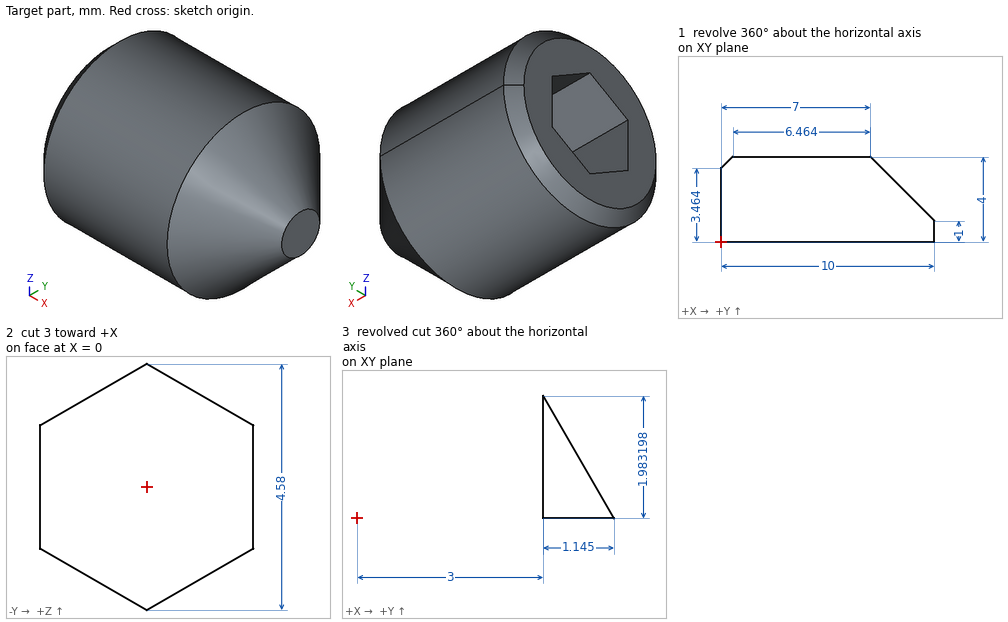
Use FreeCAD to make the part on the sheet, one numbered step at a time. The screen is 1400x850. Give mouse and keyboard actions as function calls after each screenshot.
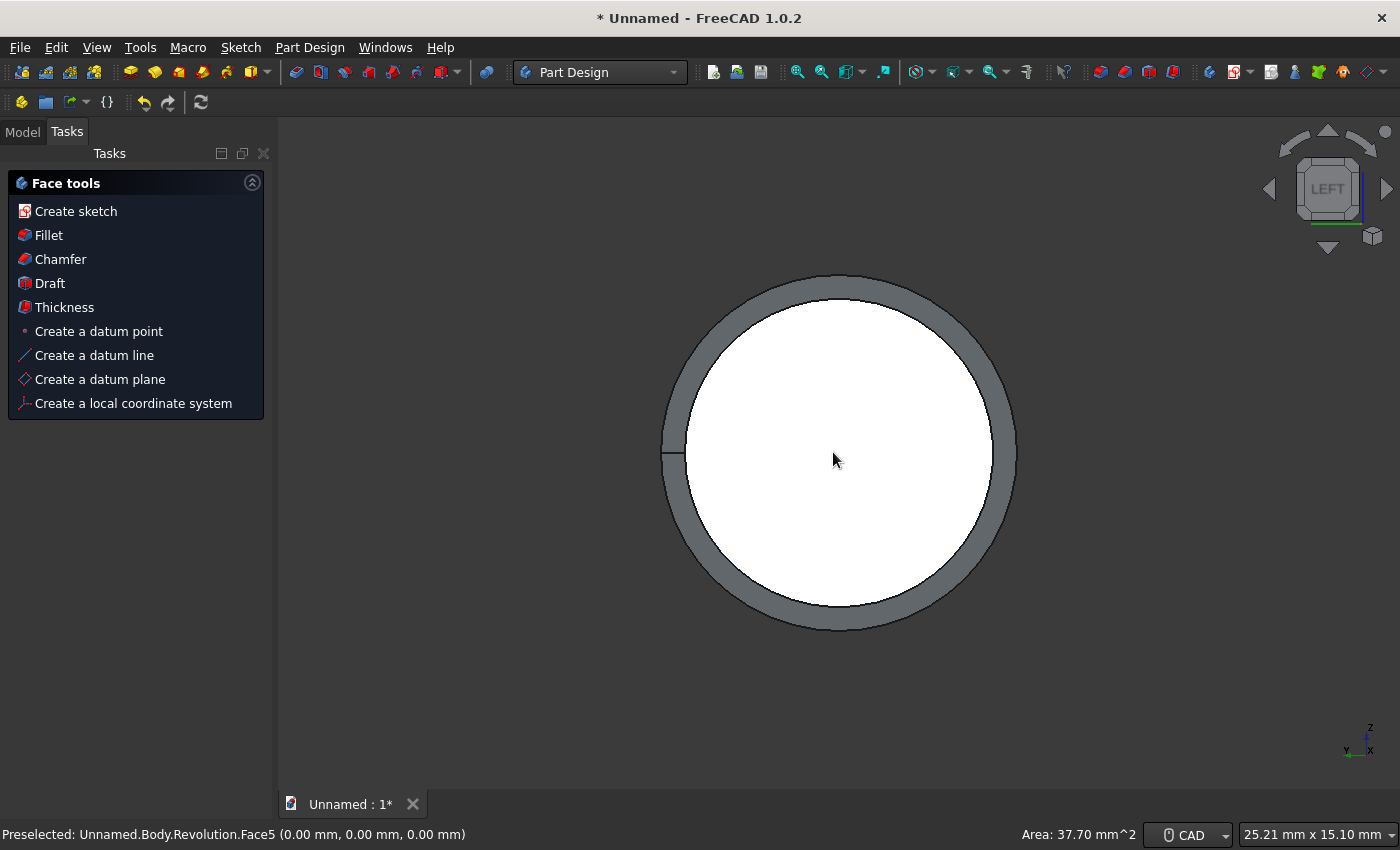
click(1234, 72)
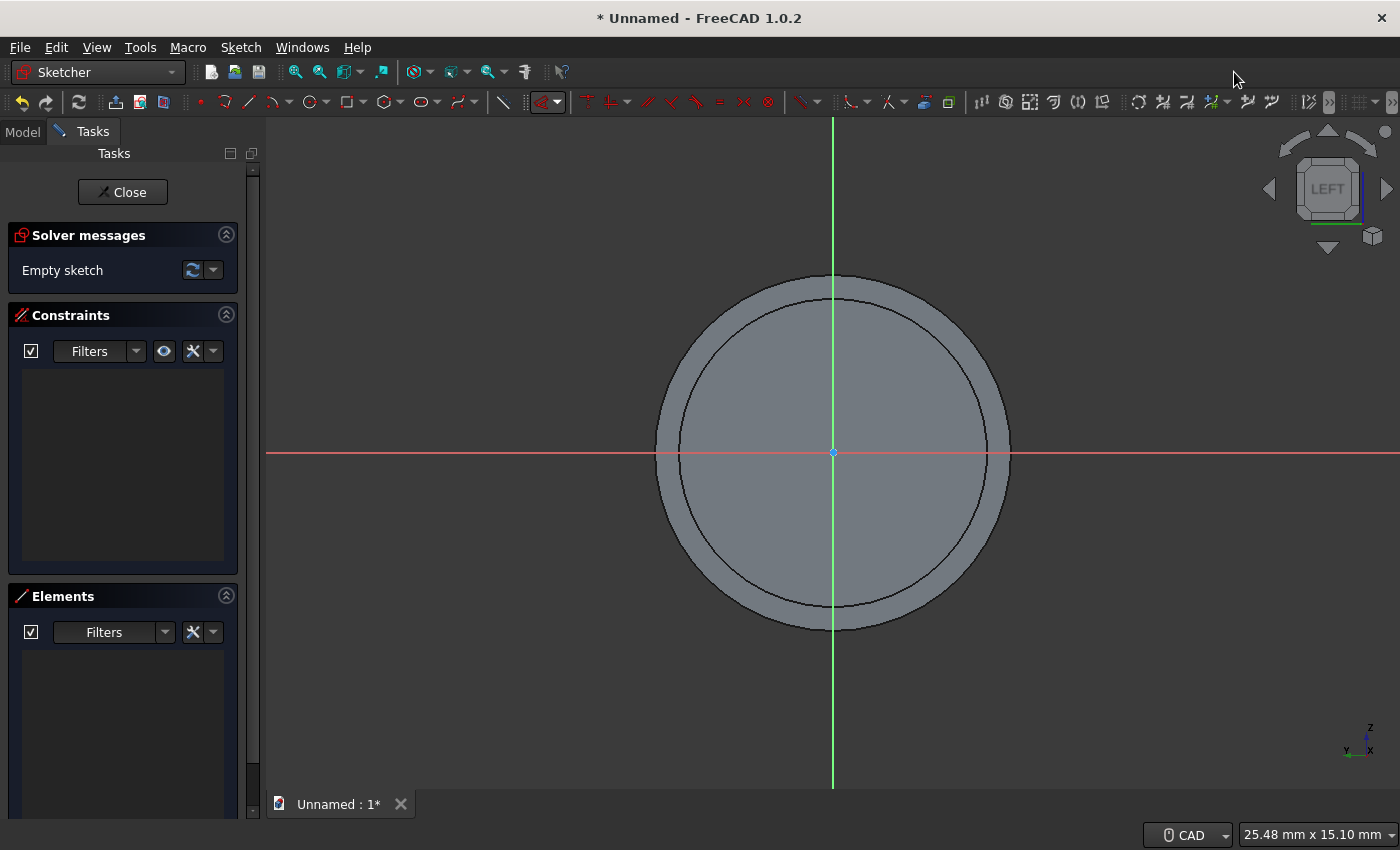
scroll(889, 453, up, 4)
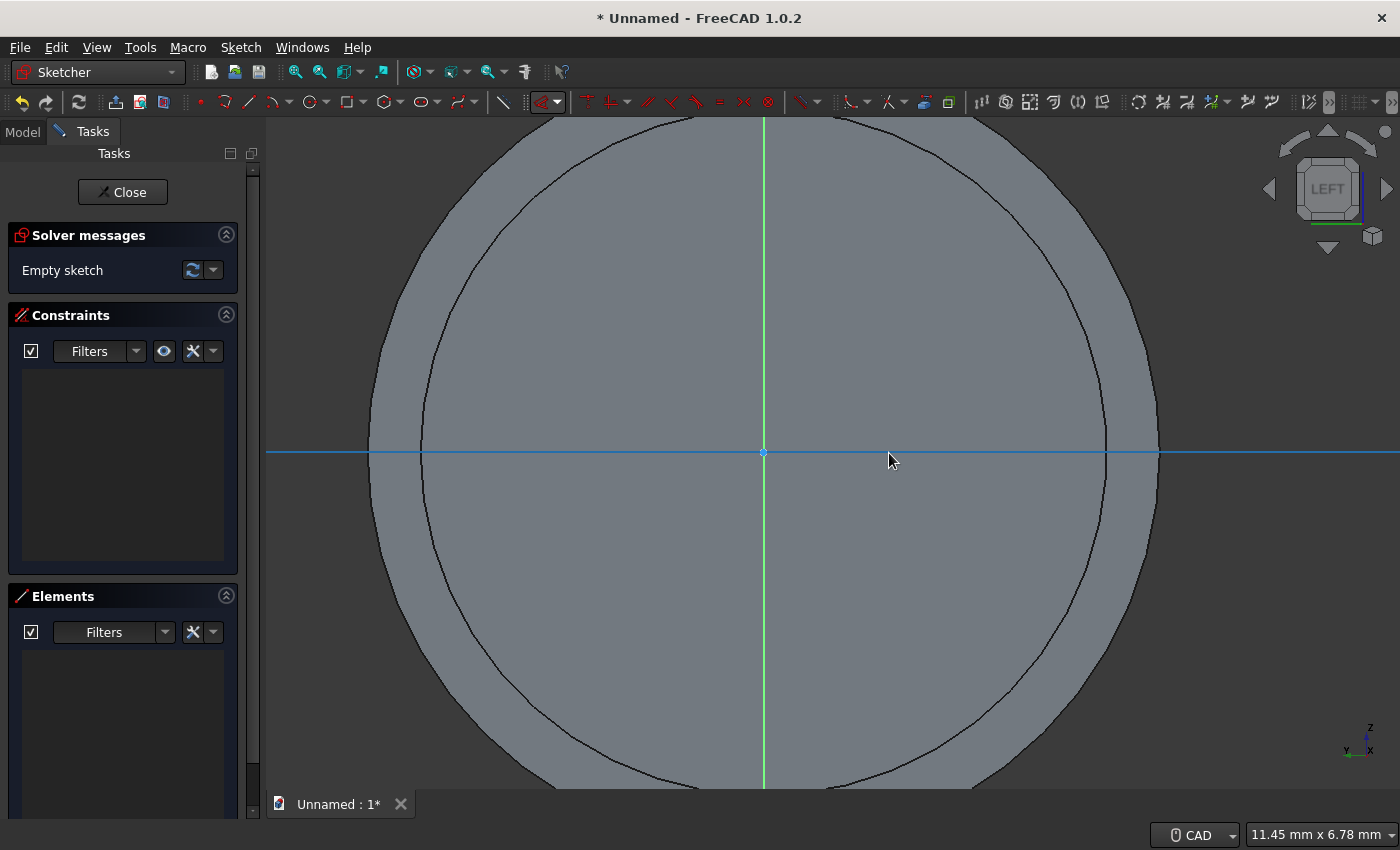
click(384, 102)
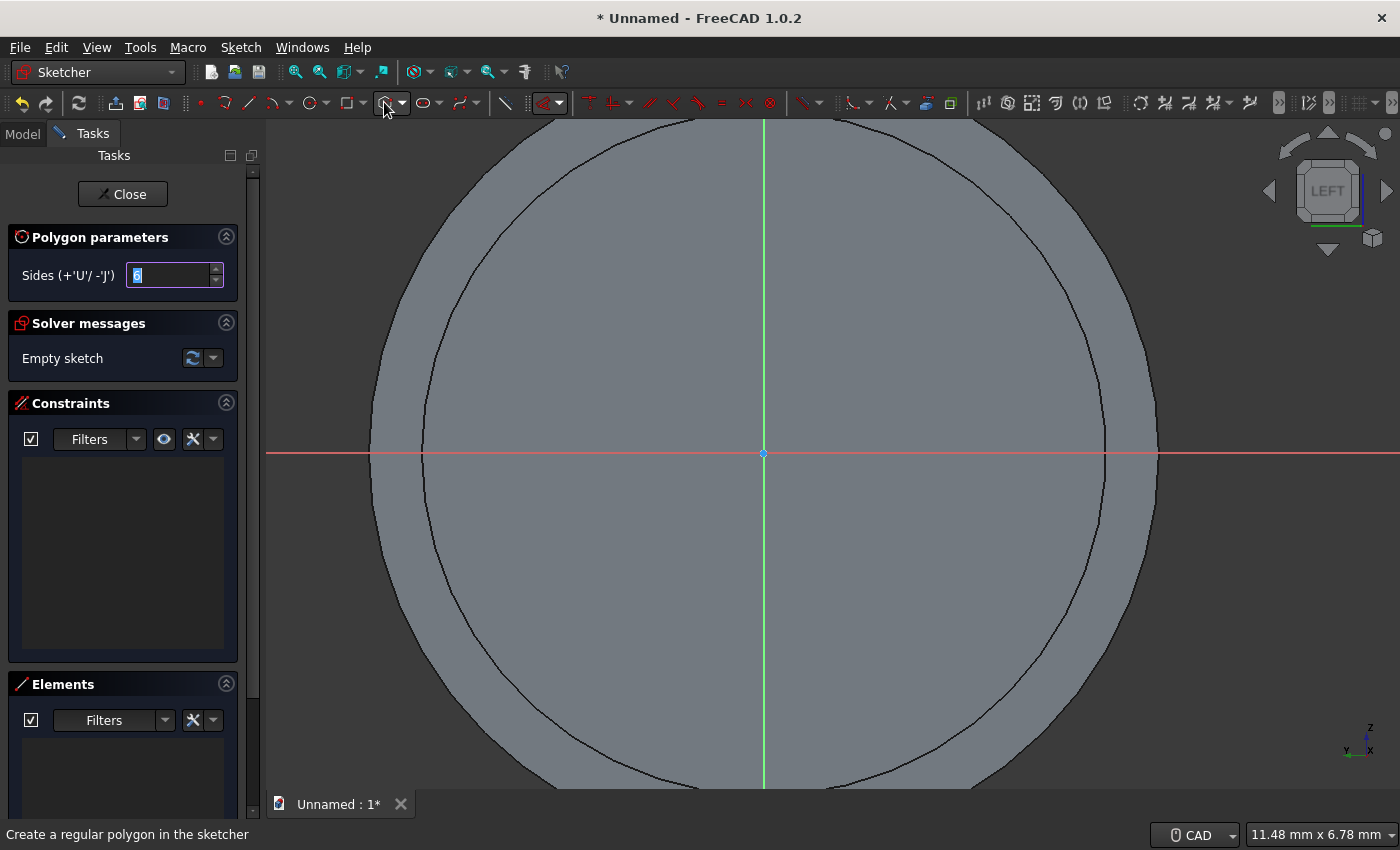
click(764, 453)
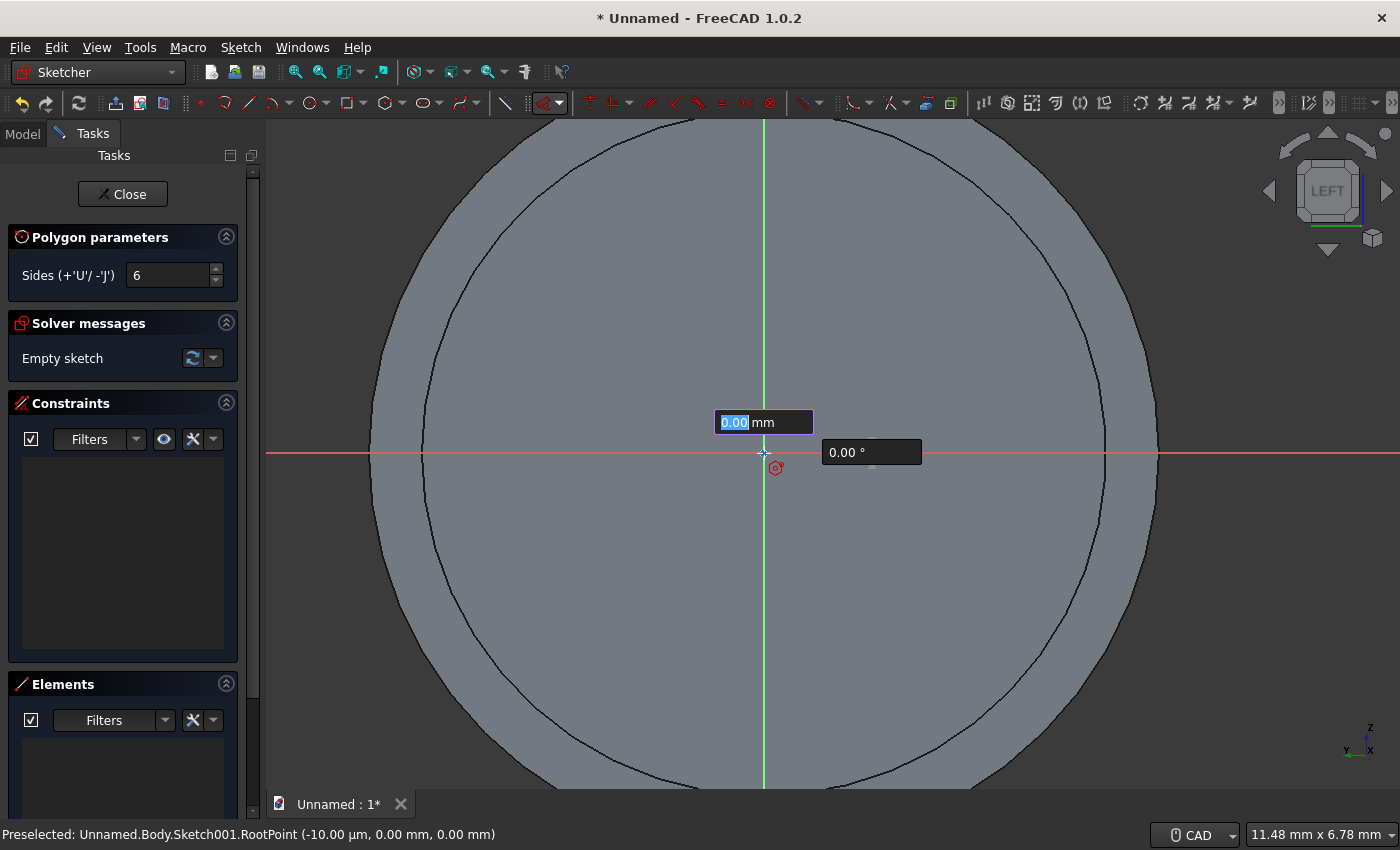
click(764, 227)
right_click(764, 227)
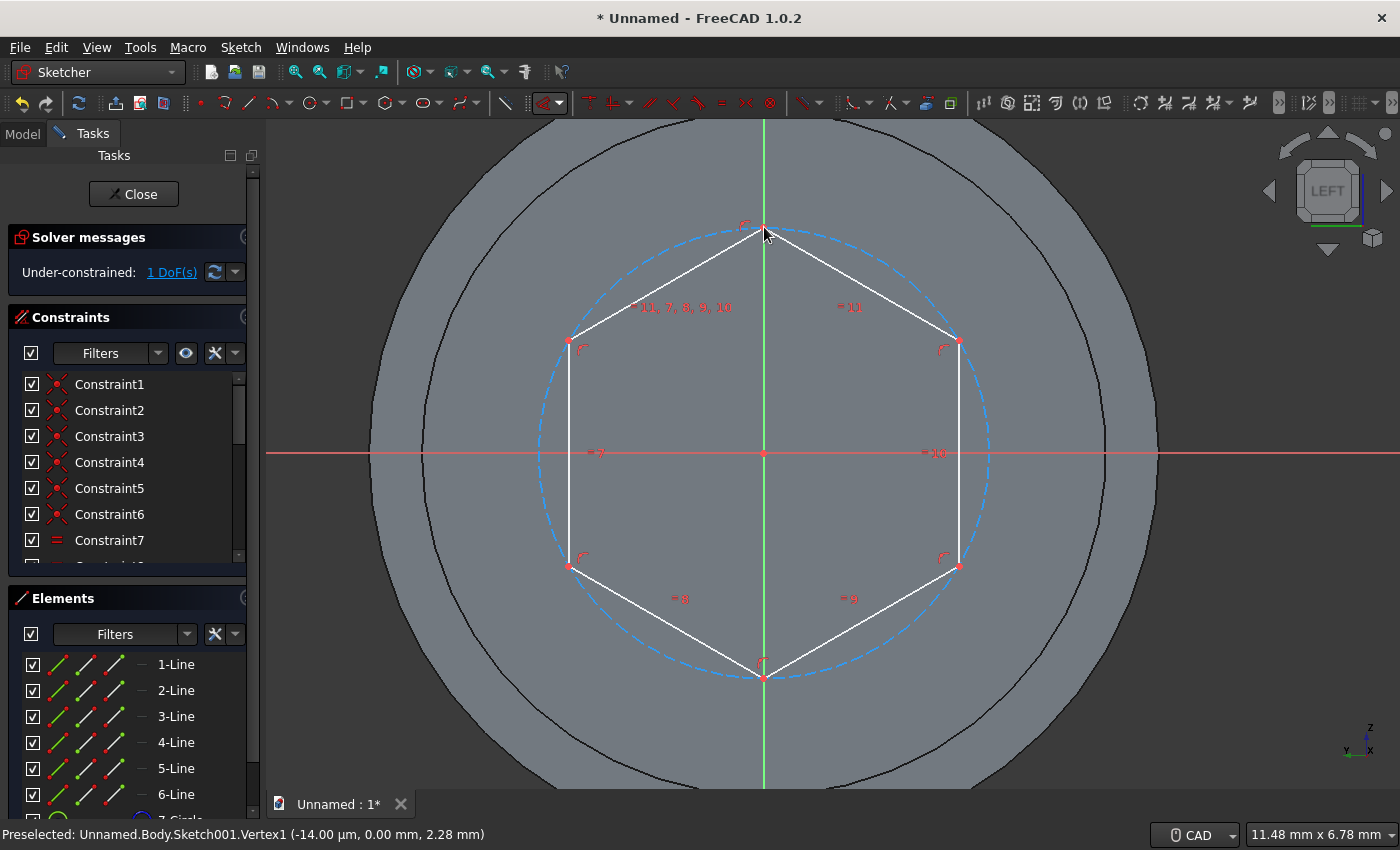
click(764, 679)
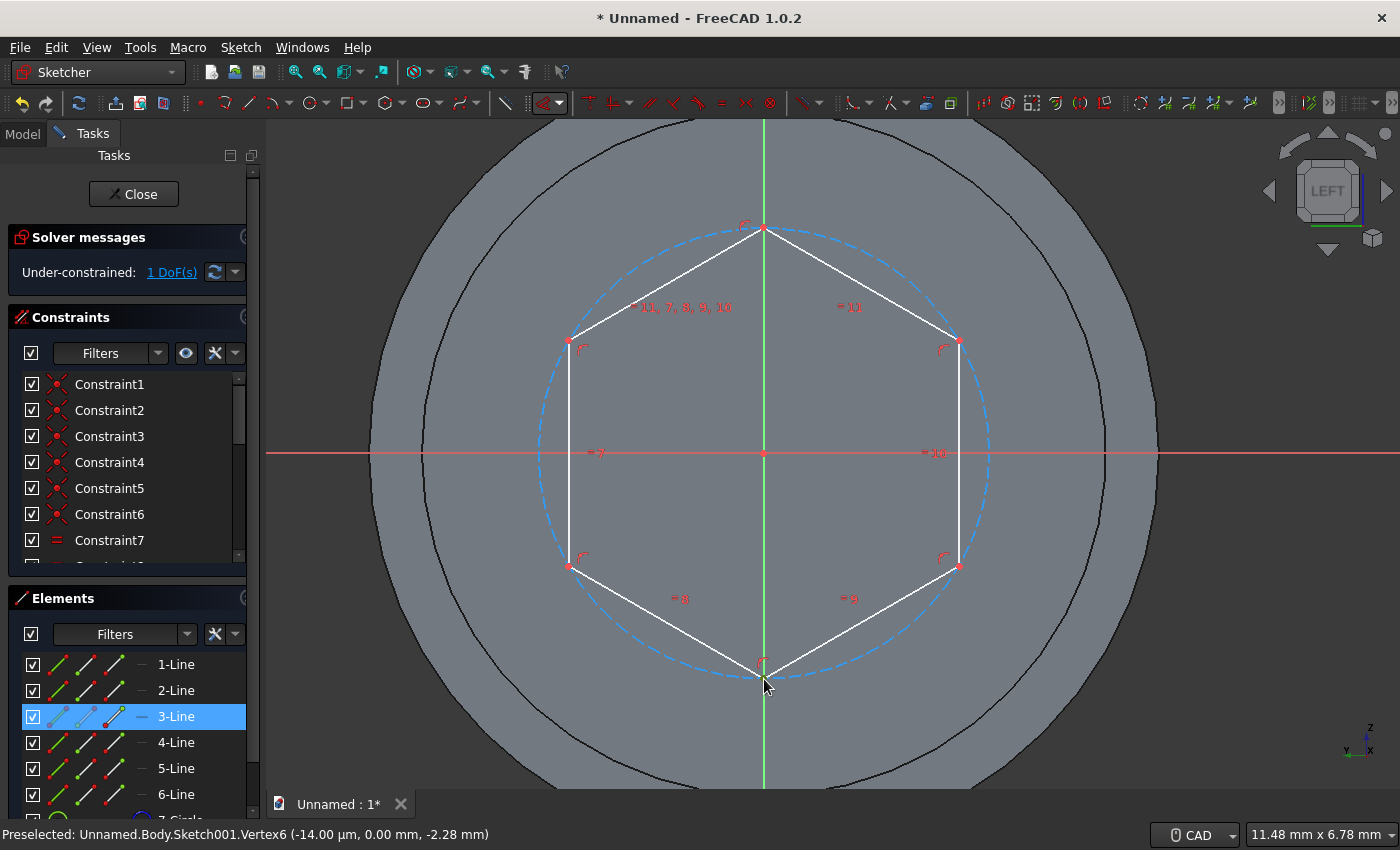
click(764, 228)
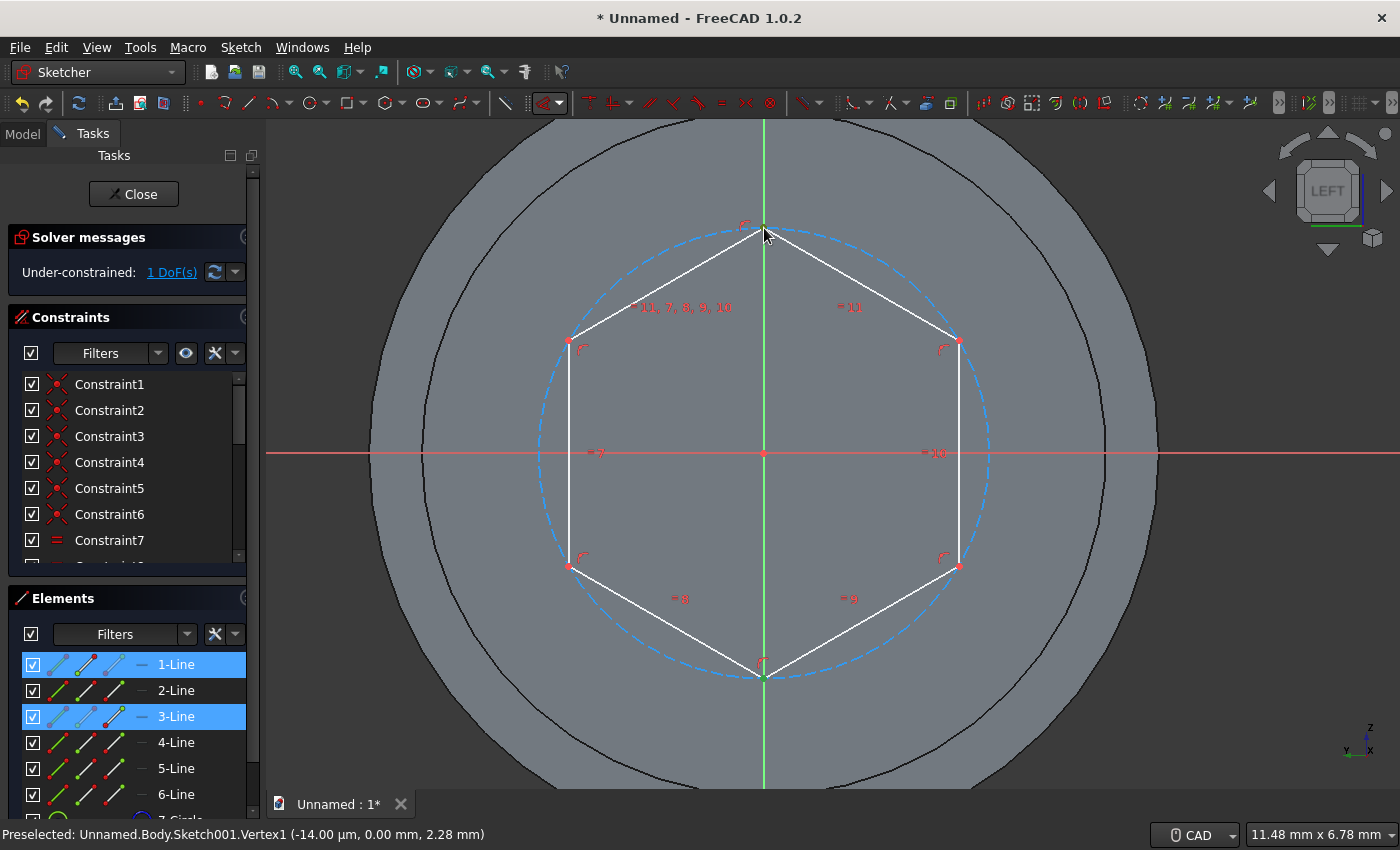
key(i)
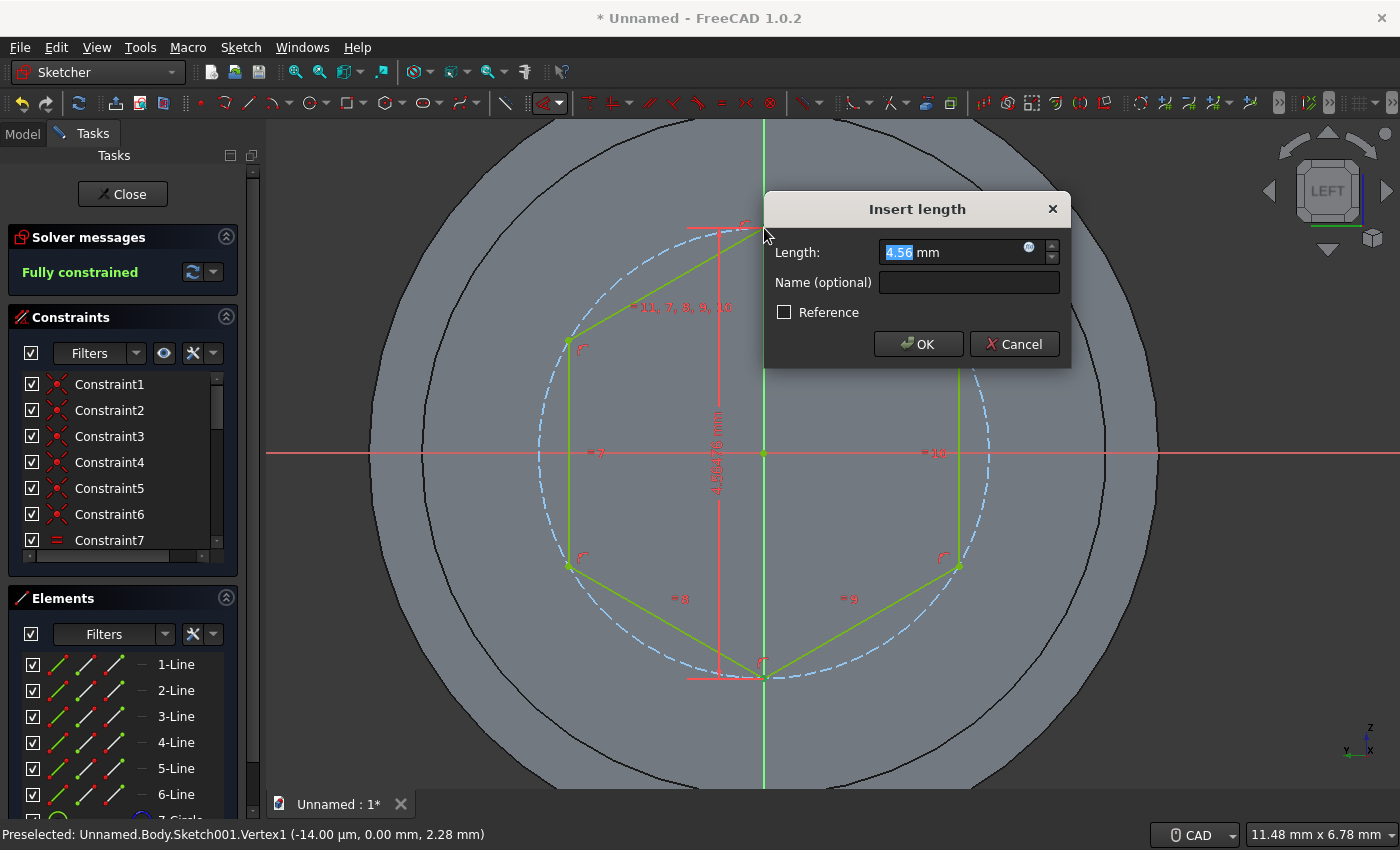
text(4.58)
key(Return)